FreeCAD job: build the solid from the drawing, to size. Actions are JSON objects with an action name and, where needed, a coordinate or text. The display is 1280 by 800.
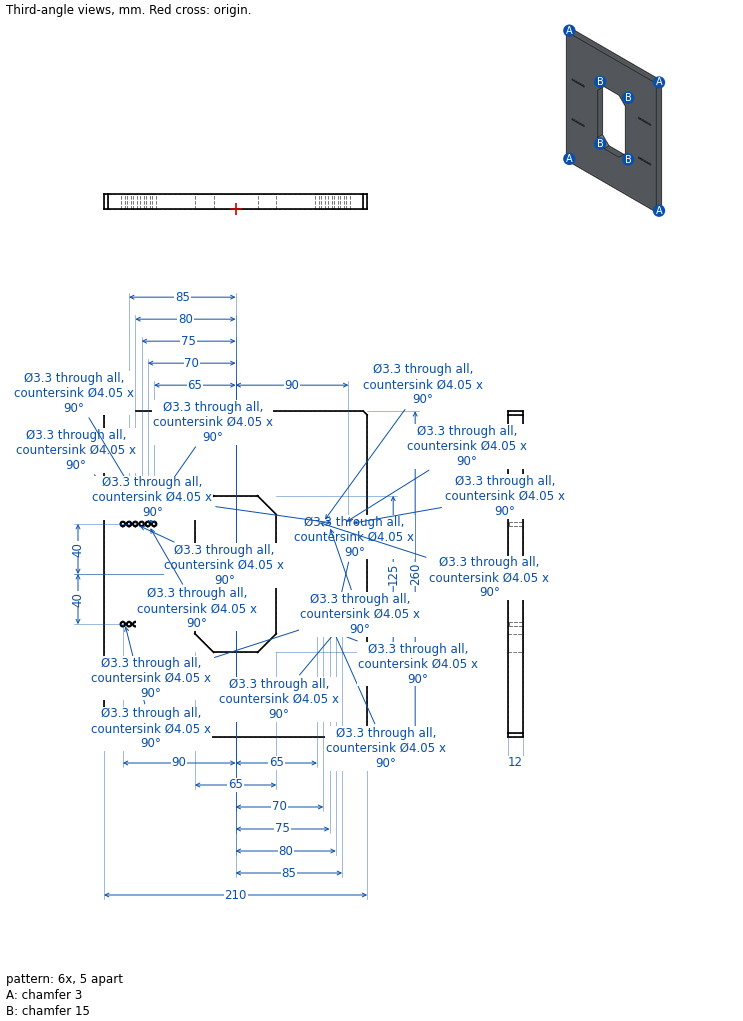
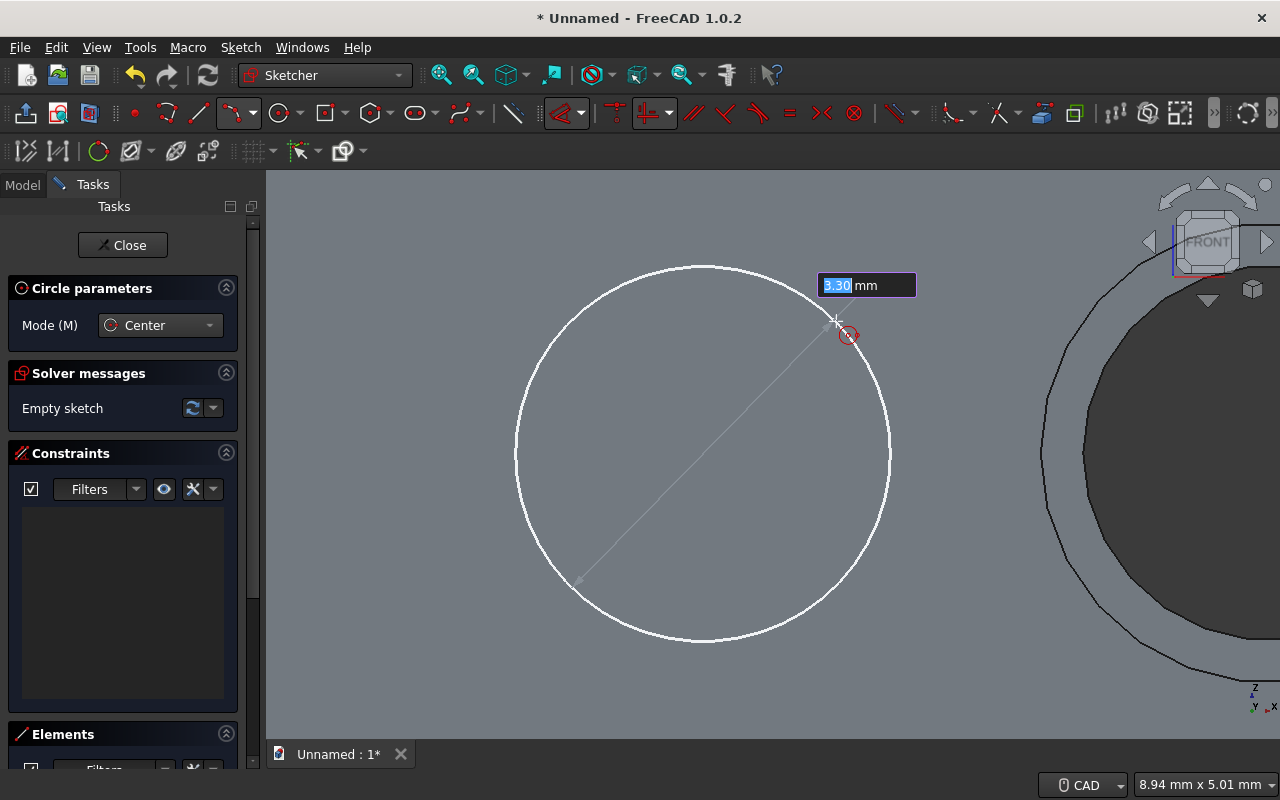
{"action": "type", "text": "3.3"}
{"action": "key", "text": "Return"}
{"action": "key", "text": "Escape"}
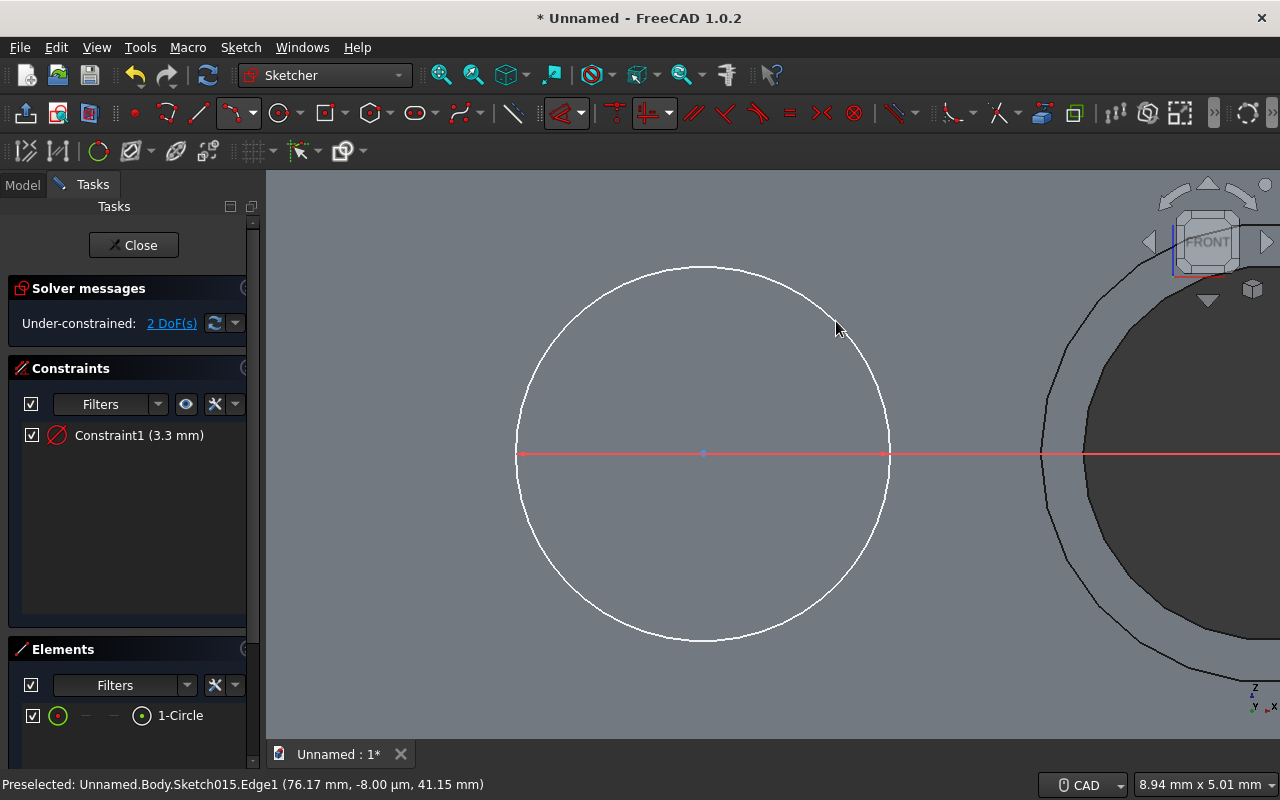
{"action": "left_click", "coordinate": [703, 454]}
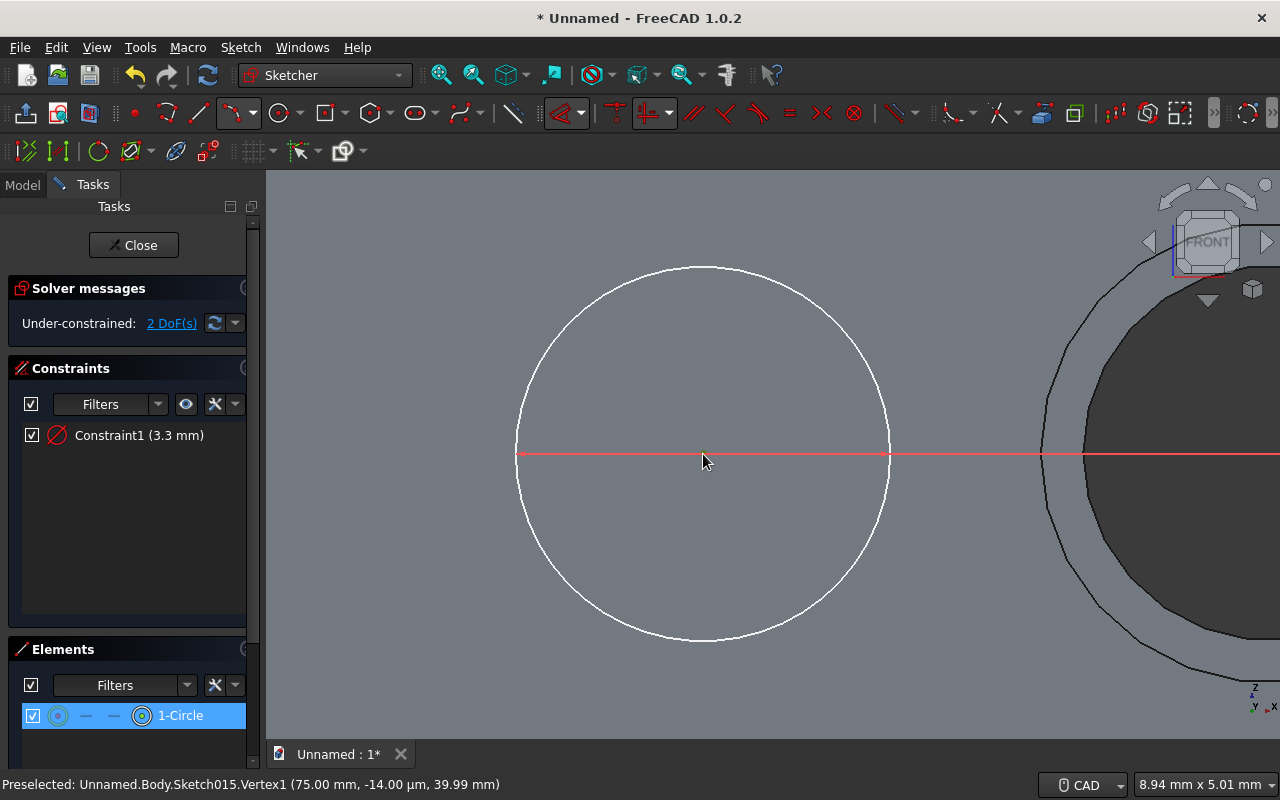
{"action": "left_click", "coordinate": [584, 114]}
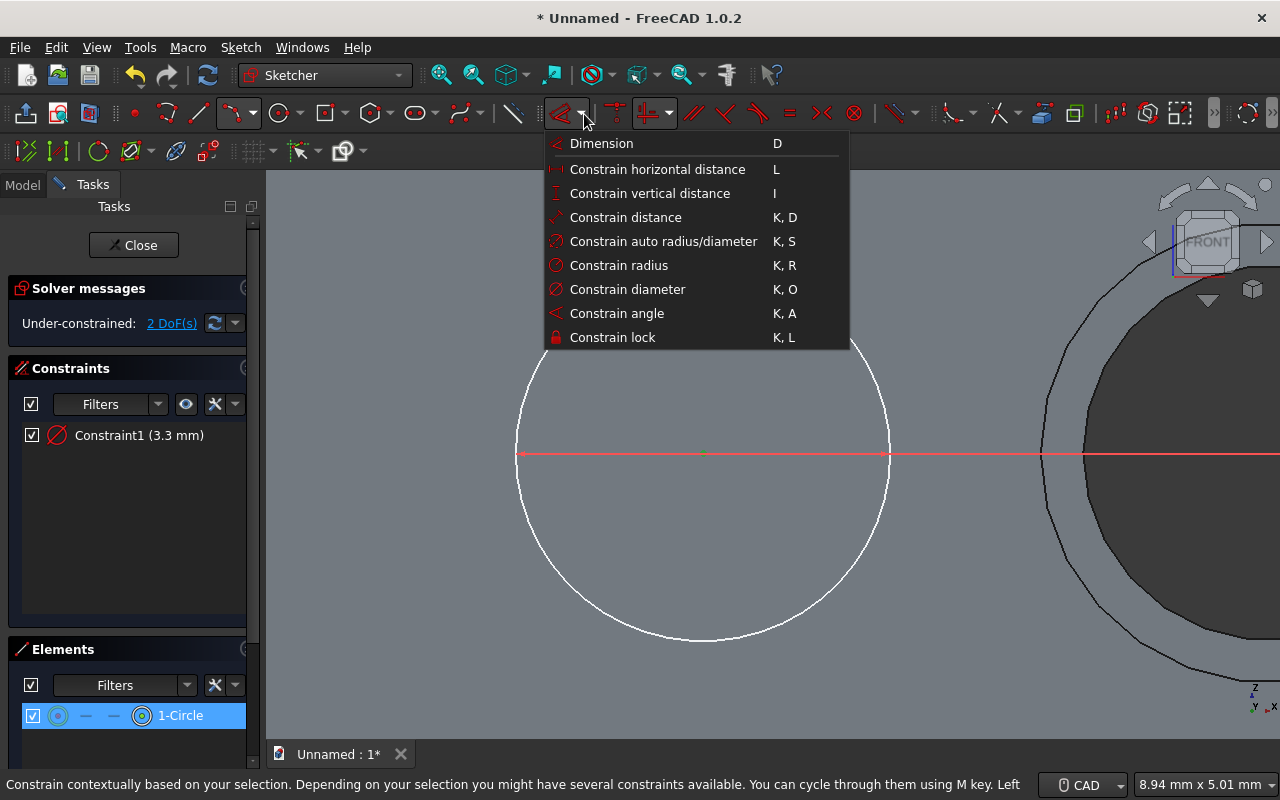
{"action": "left_click", "coordinate": [697, 169]}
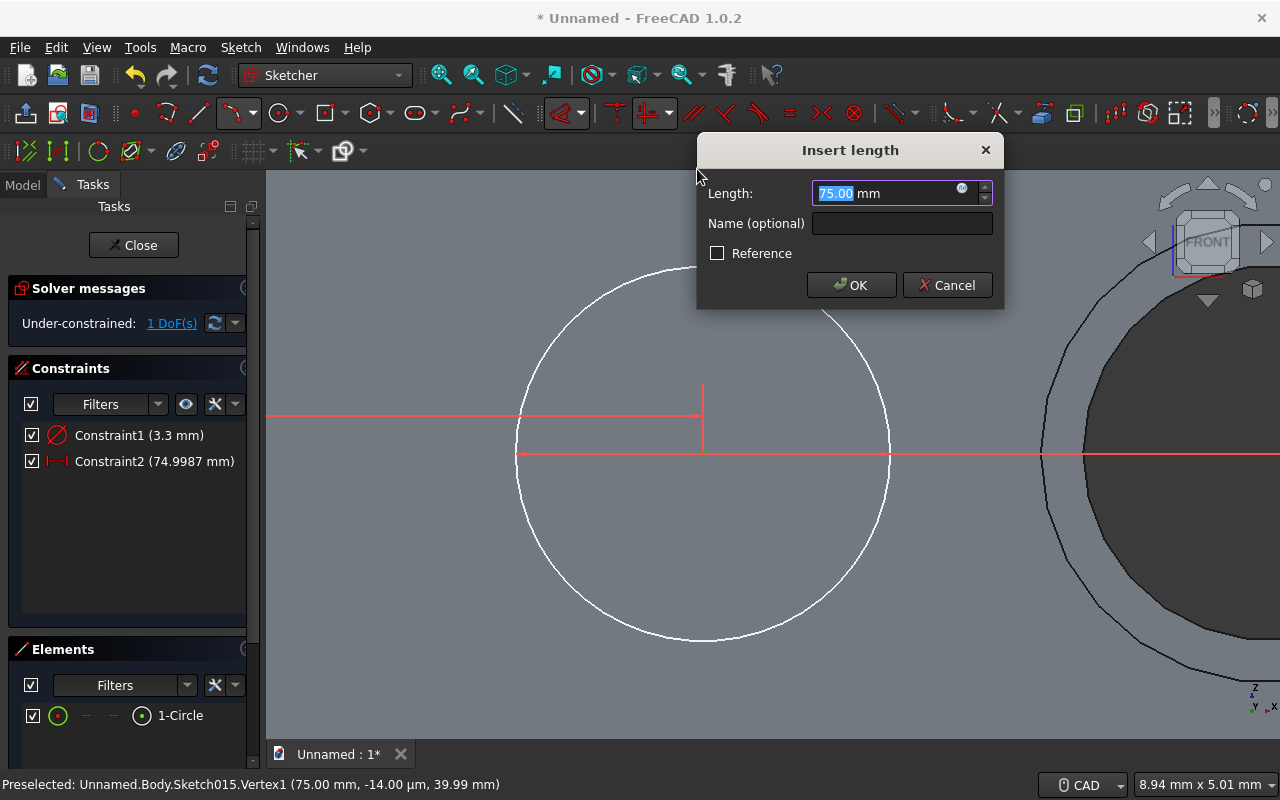
{"action": "type", "text": "75"}
{"action": "key", "text": "Return"}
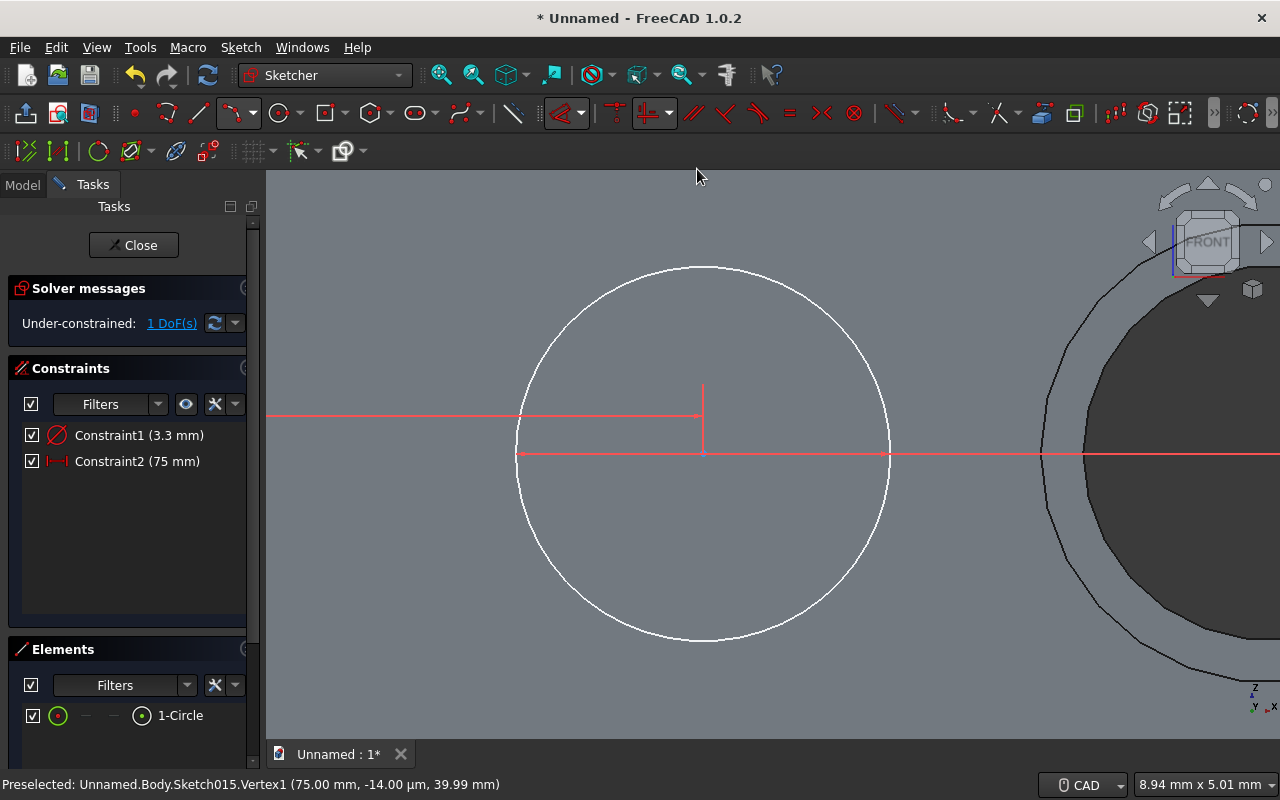
{"action": "left_click", "coordinate": [703, 454]}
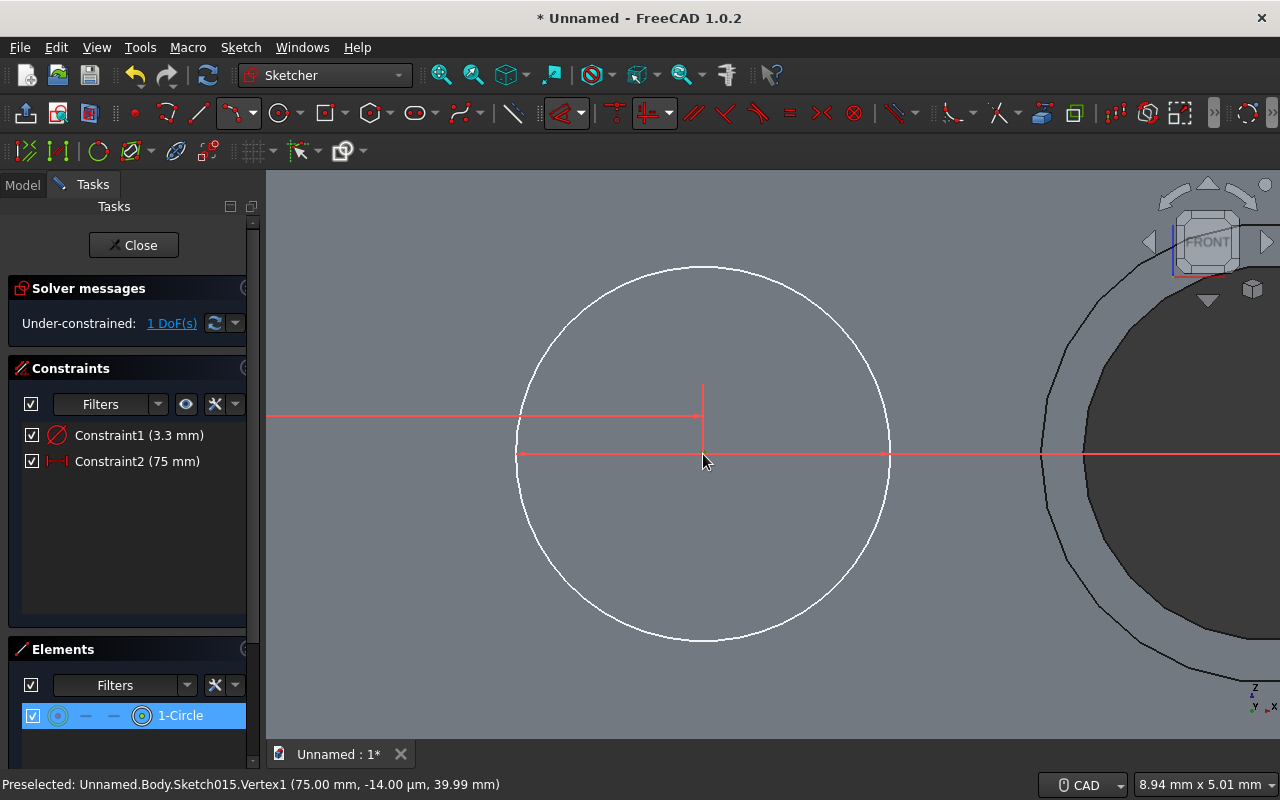
{"action": "left_click", "coordinate": [584, 114]}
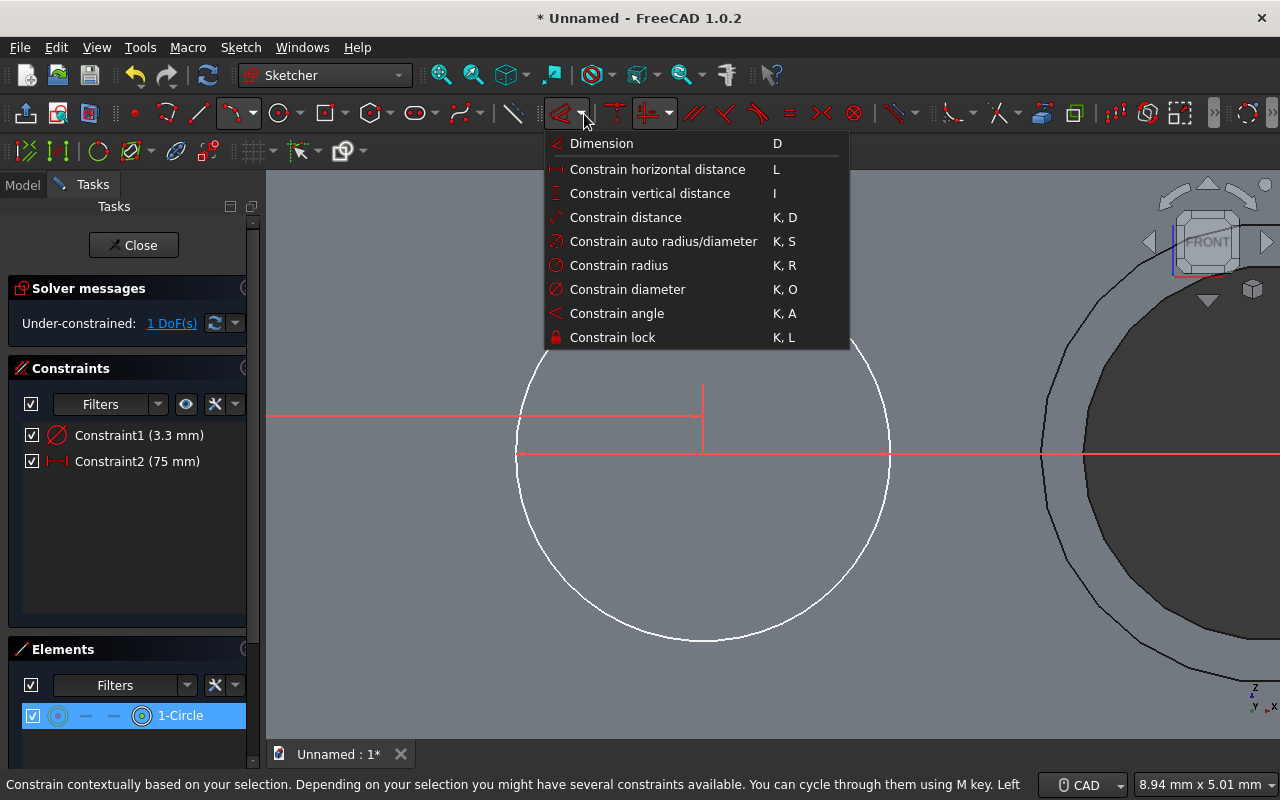
{"action": "left_click", "coordinate": [697, 193]}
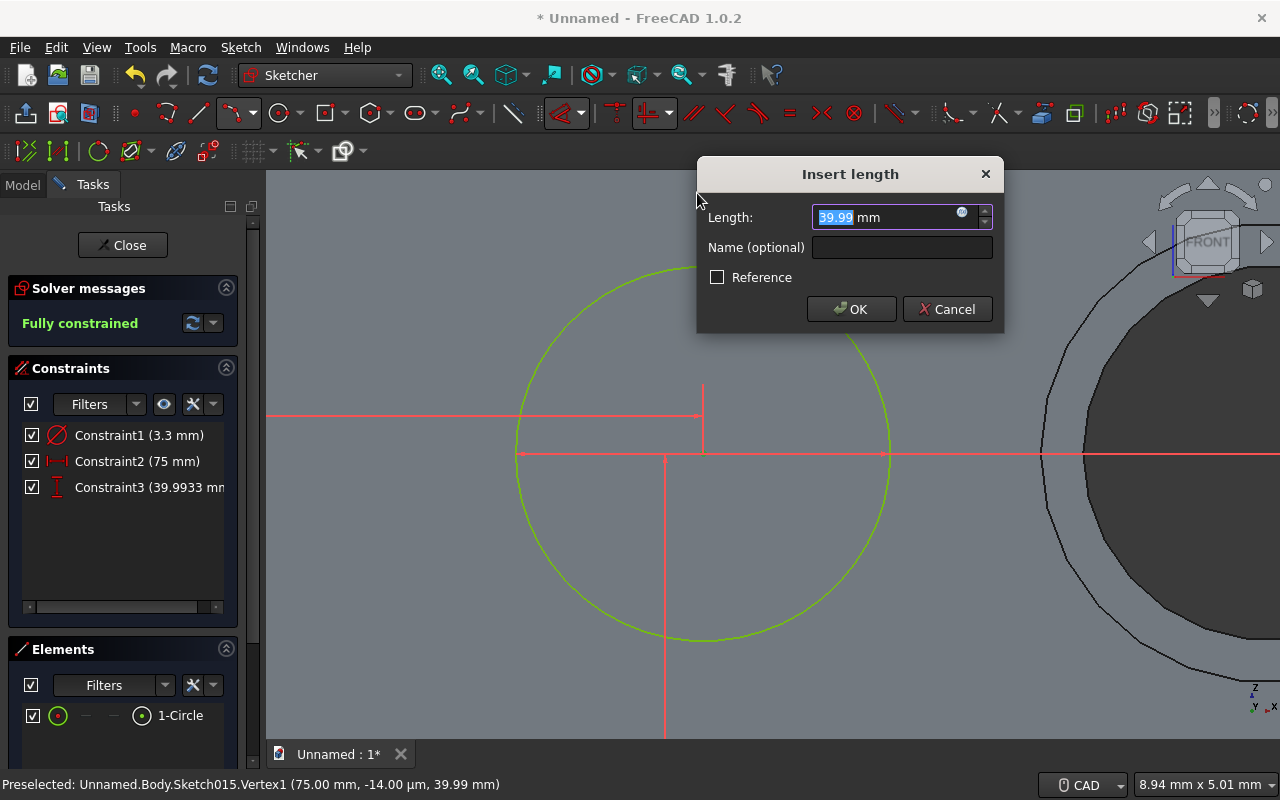
{"action": "type", "text": "40"}
{"action": "key", "text": "Return"}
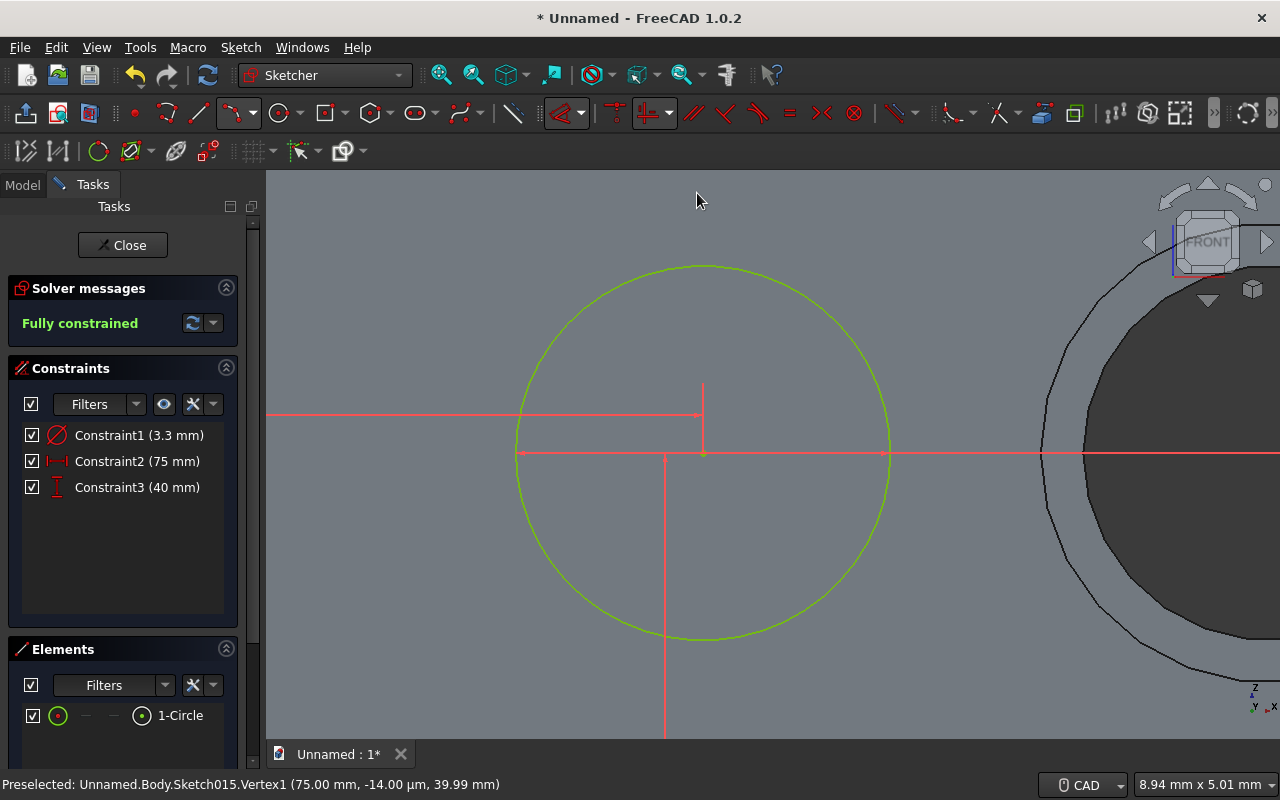
{"action": "left_click", "coordinate": [123, 245]}